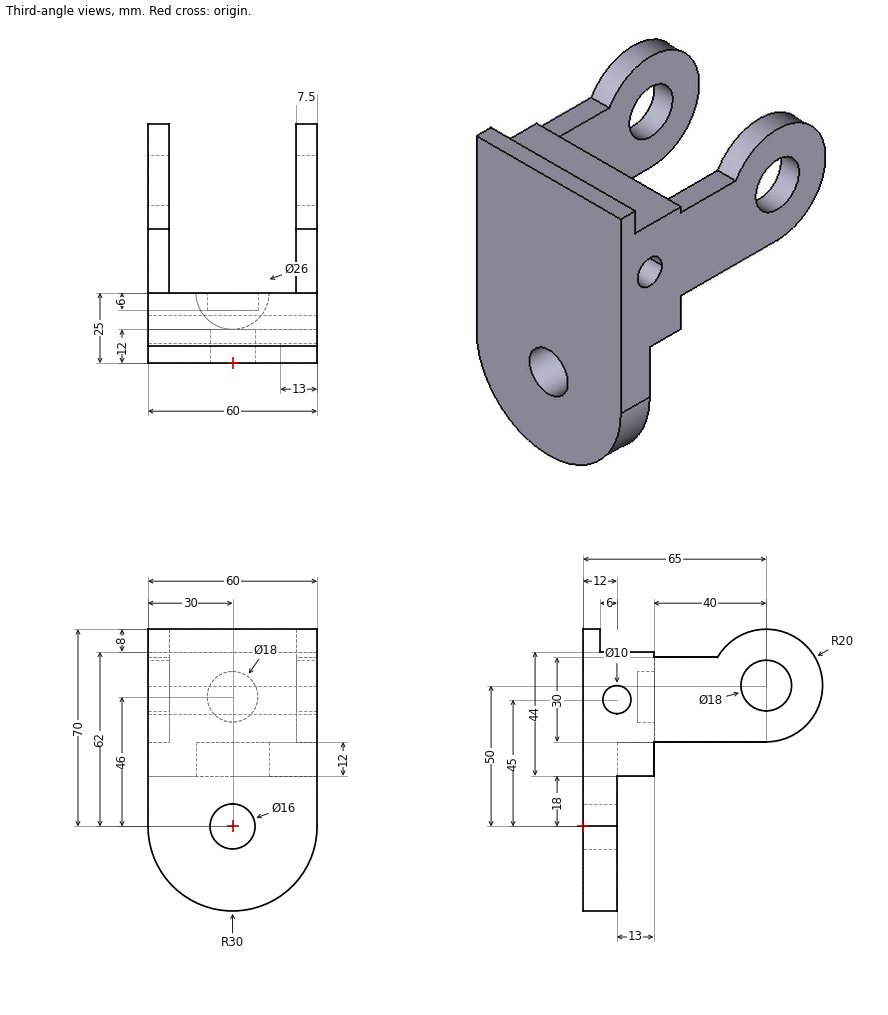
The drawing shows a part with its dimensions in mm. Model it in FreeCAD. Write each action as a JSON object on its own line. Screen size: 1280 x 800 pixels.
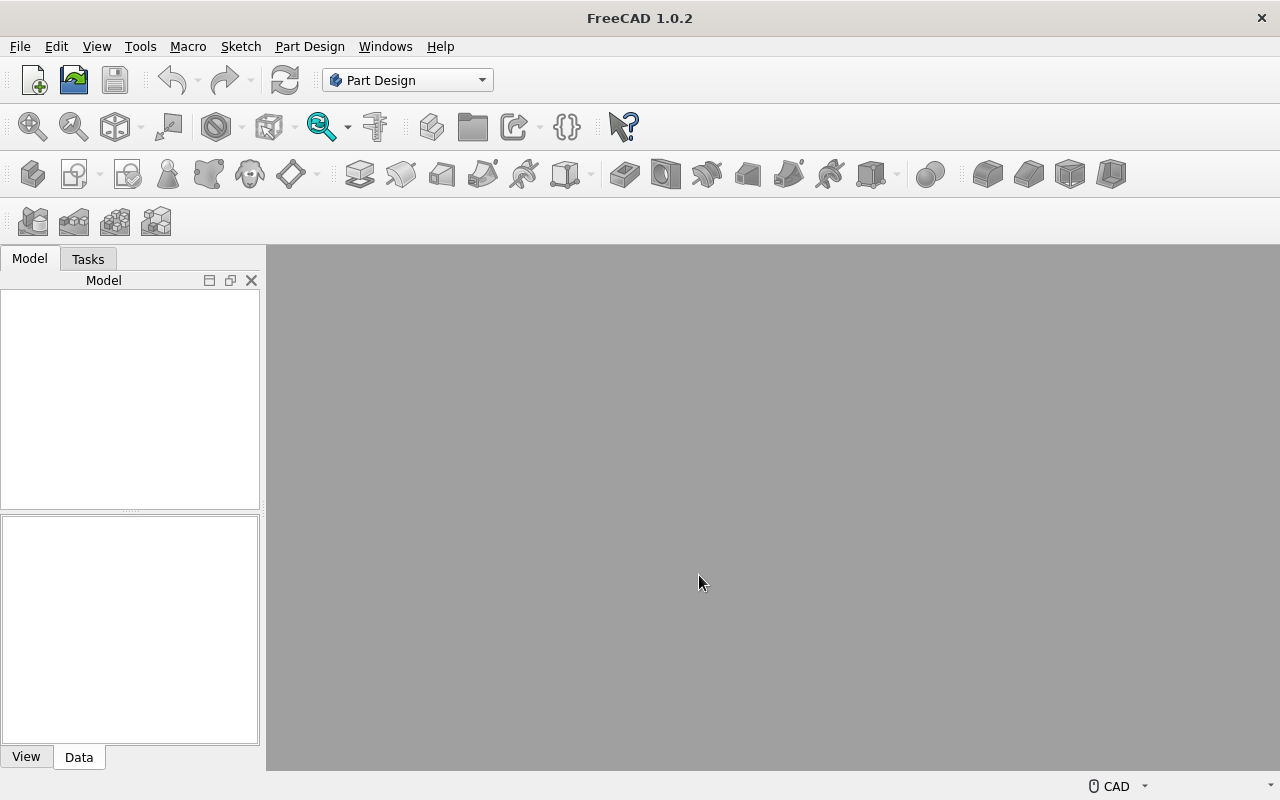
{"action": "key", "text": "ctrl+n"}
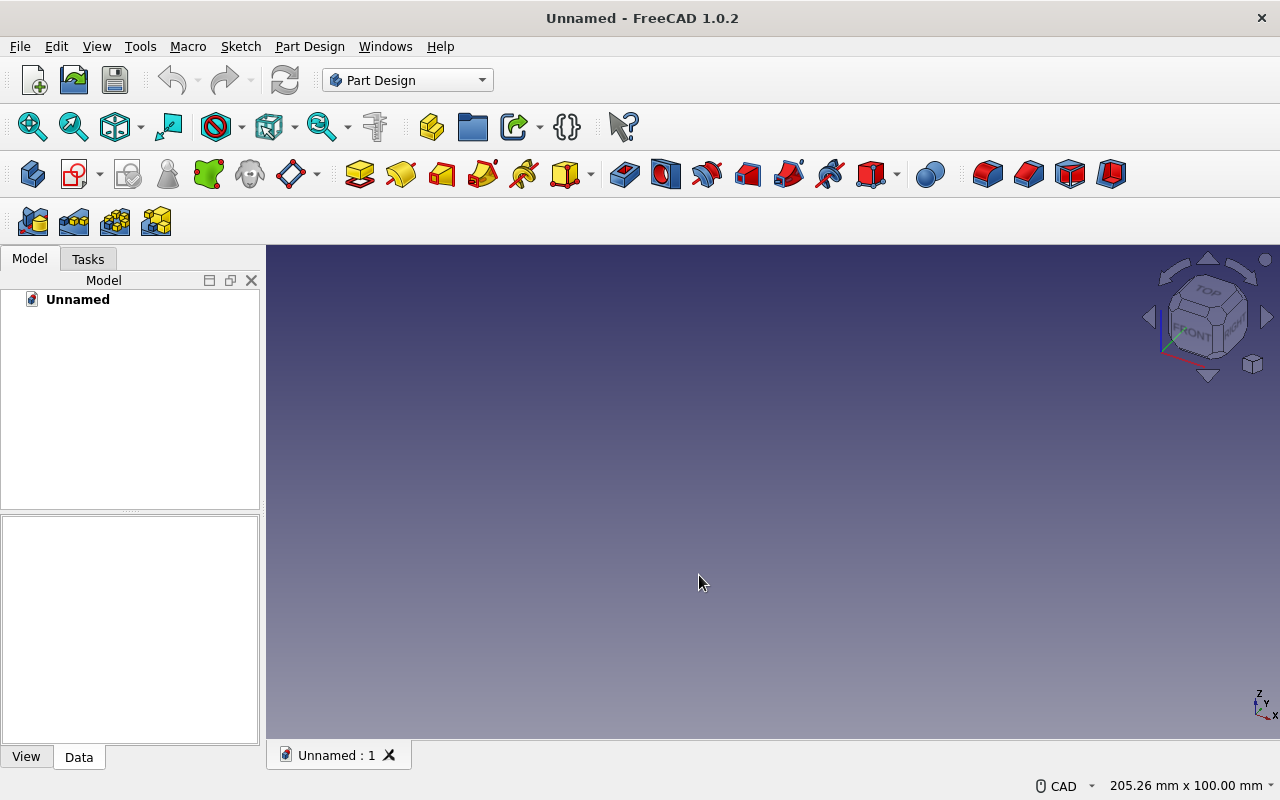
{"action": "left_click", "coordinate": [74, 174]}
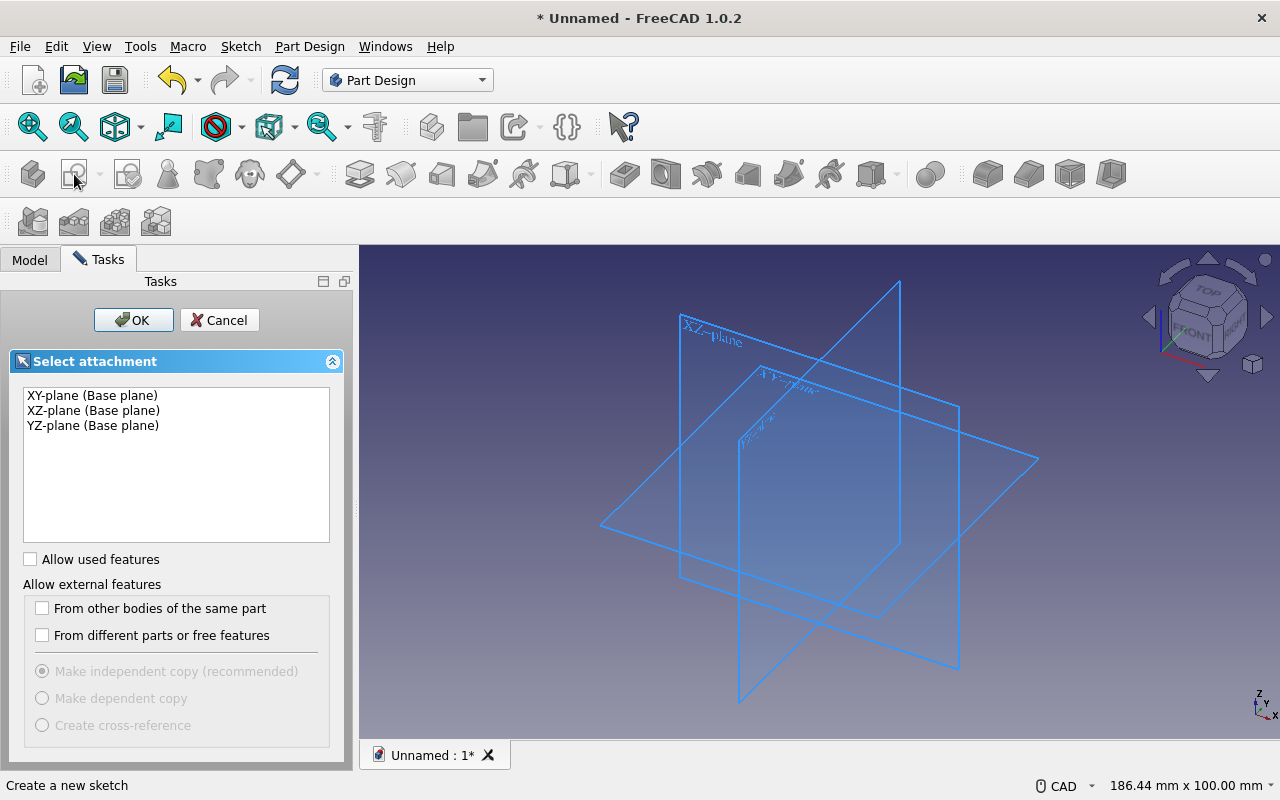
{"action": "left_click", "coordinate": [84, 410]}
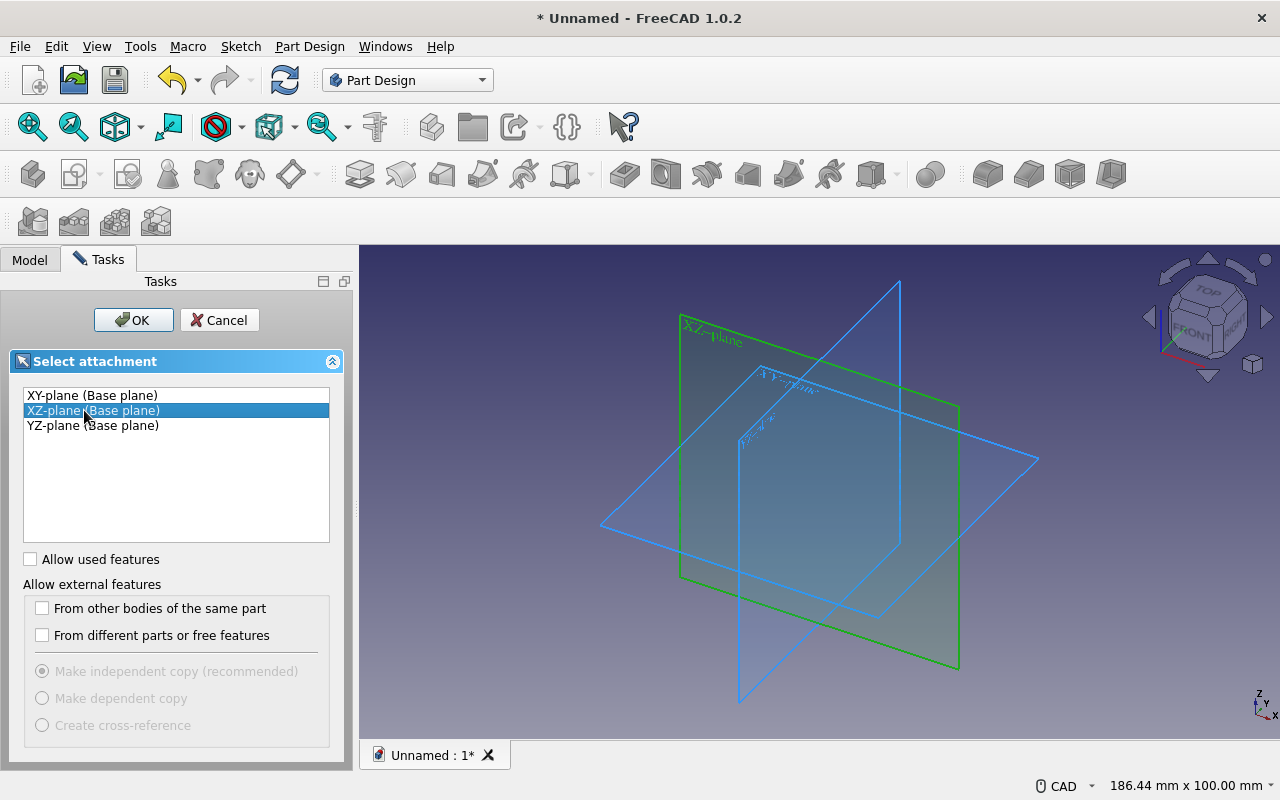
{"action": "left_click", "coordinate": [134, 320]}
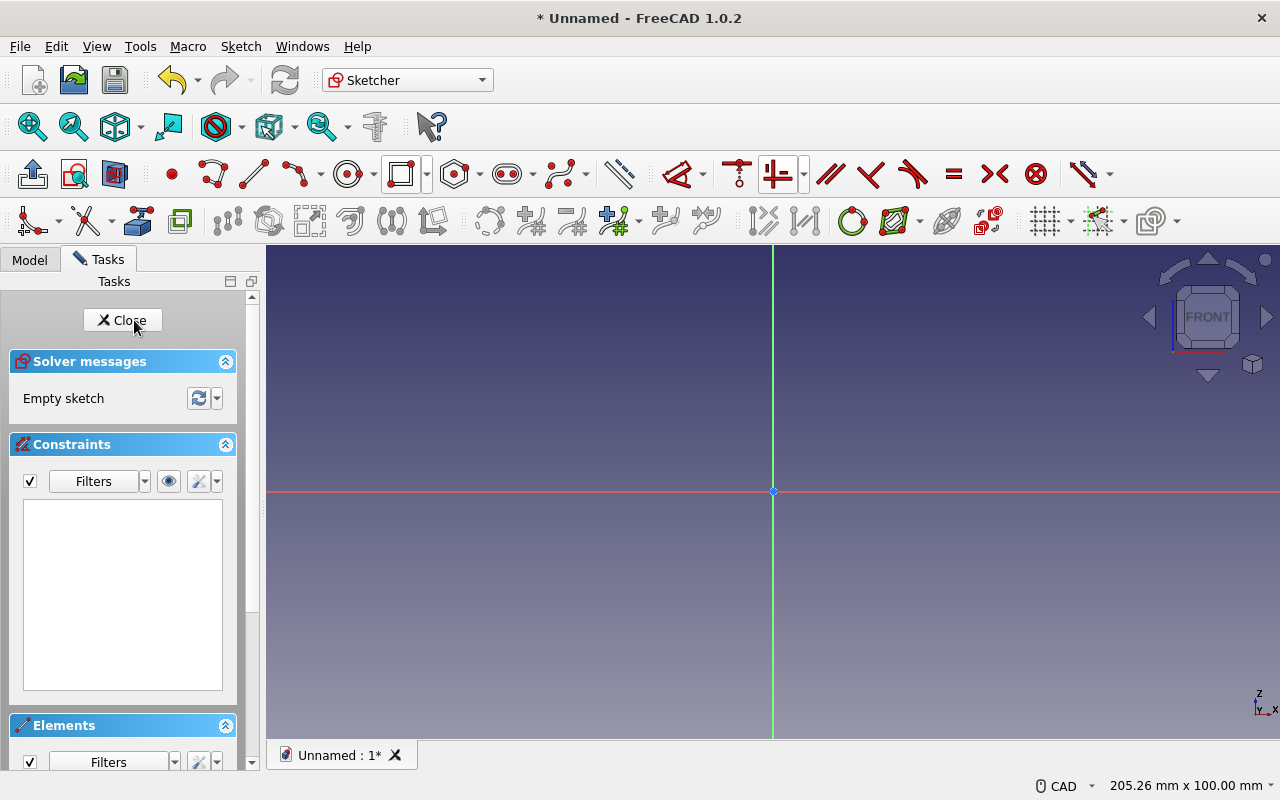
{"action": "scroll", "coordinate": [565, 693], "scroll_direction": "down", "scroll_amount": 2}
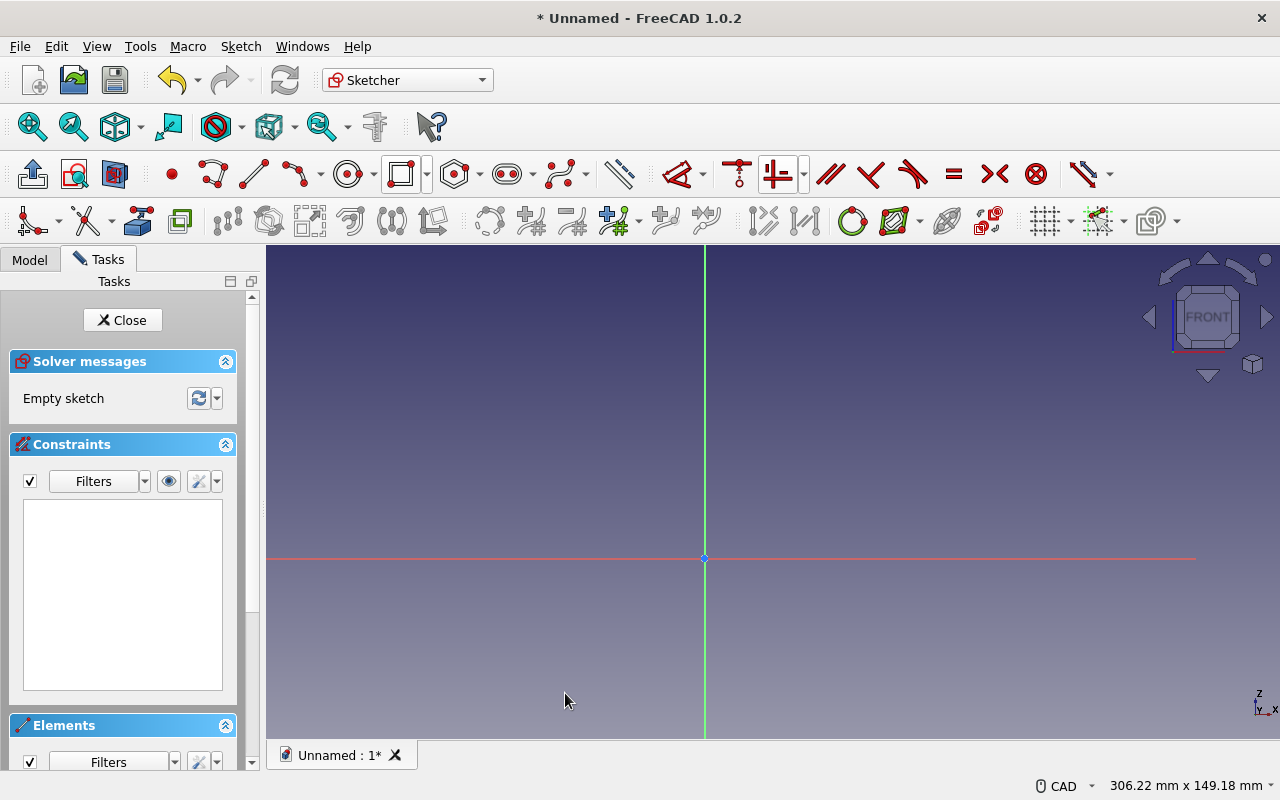
{"action": "left_click", "coordinate": [213, 174]}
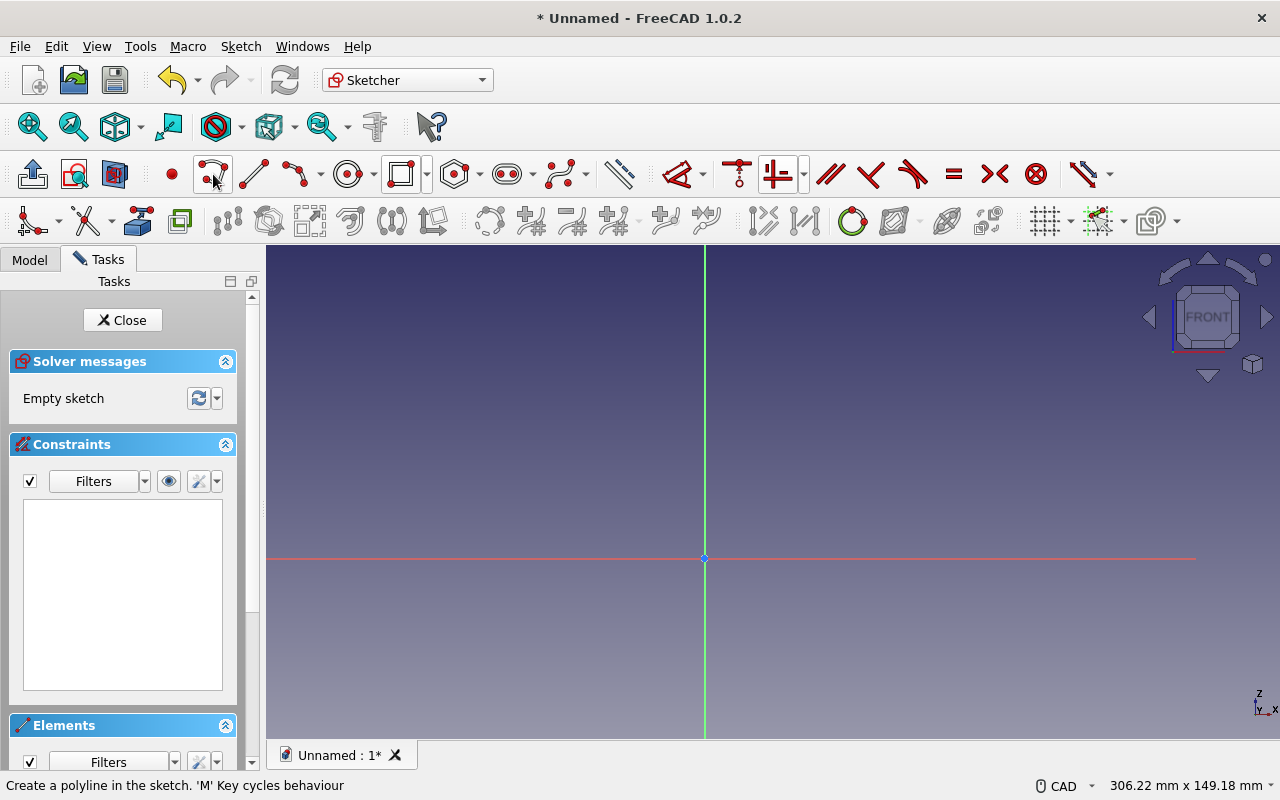
{"action": "left_click", "coordinate": [605, 559]}
{"action": "left_click", "coordinate": [605, 327]}
{"action": "left_click", "coordinate": [804, 327]}
{"action": "left_click", "coordinate": [804, 559]}
{"action": "right_click", "coordinate": [804, 559]}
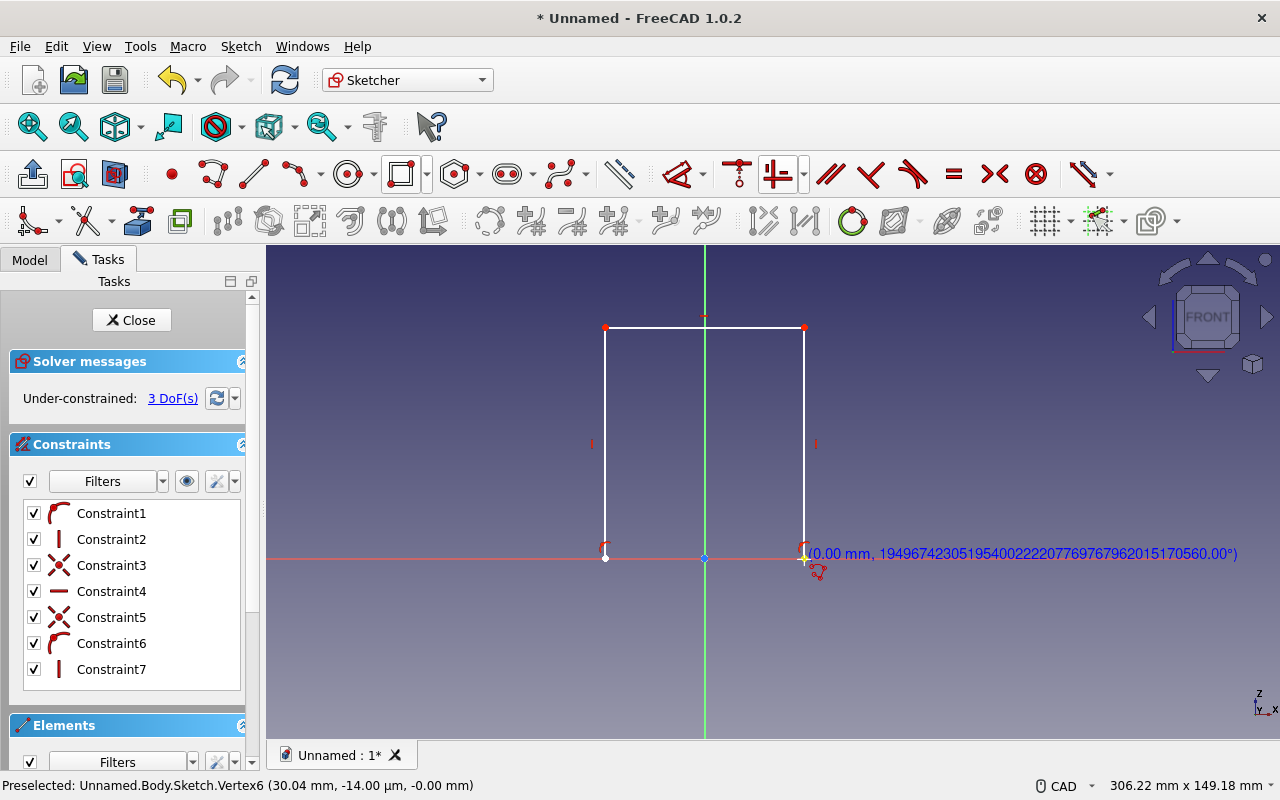
{"action": "left_click", "coordinate": [294, 174]}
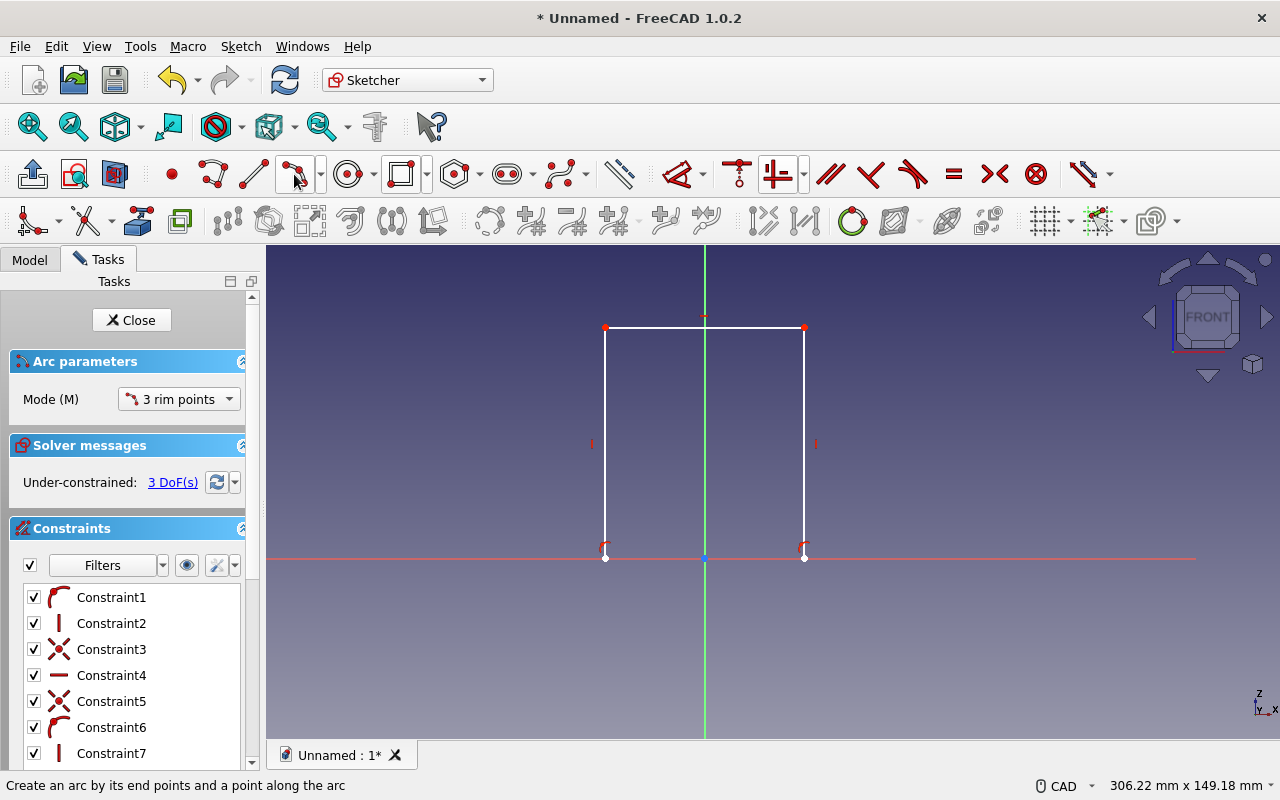
{"action": "left_click", "coordinate": [804, 559]}
{"action": "left_click", "coordinate": [605, 559]}
{"action": "left_click", "coordinate": [674, 653]}
{"action": "key", "text": "Escape"}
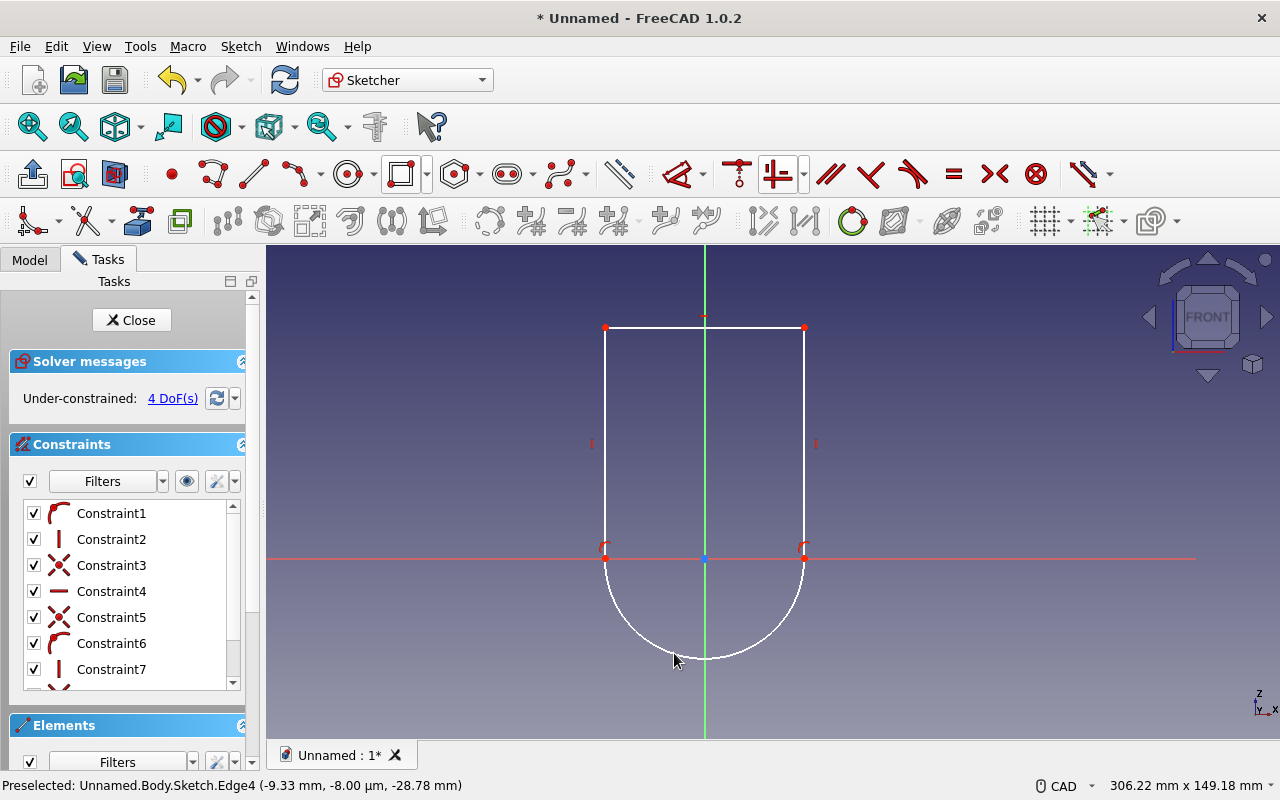
{"action": "left_click_drag", "start_coordinate": [695, 549], "coordinate": [715, 569]}